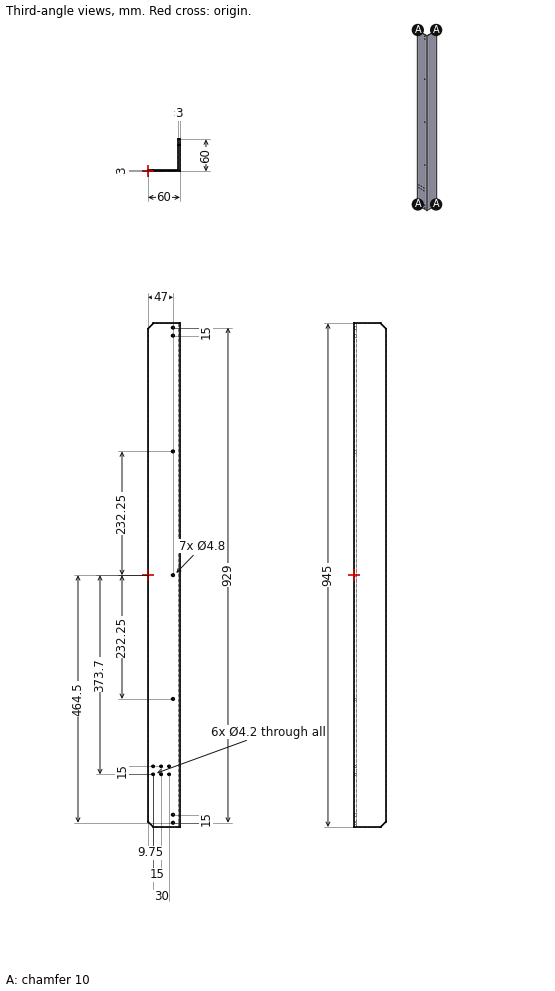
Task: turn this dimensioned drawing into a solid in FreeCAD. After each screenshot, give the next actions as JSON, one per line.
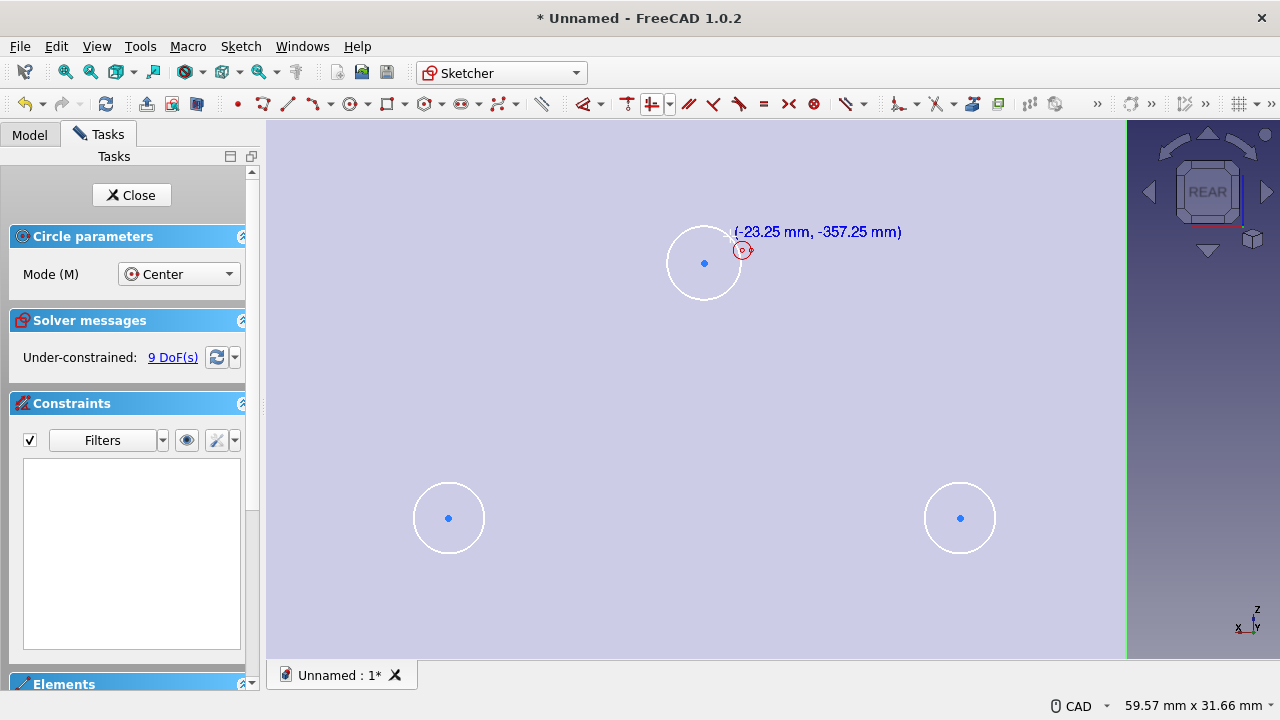
{"action": "left_click", "coordinate": [960, 262]}
{"action": "left_click", "coordinate": [985, 236]}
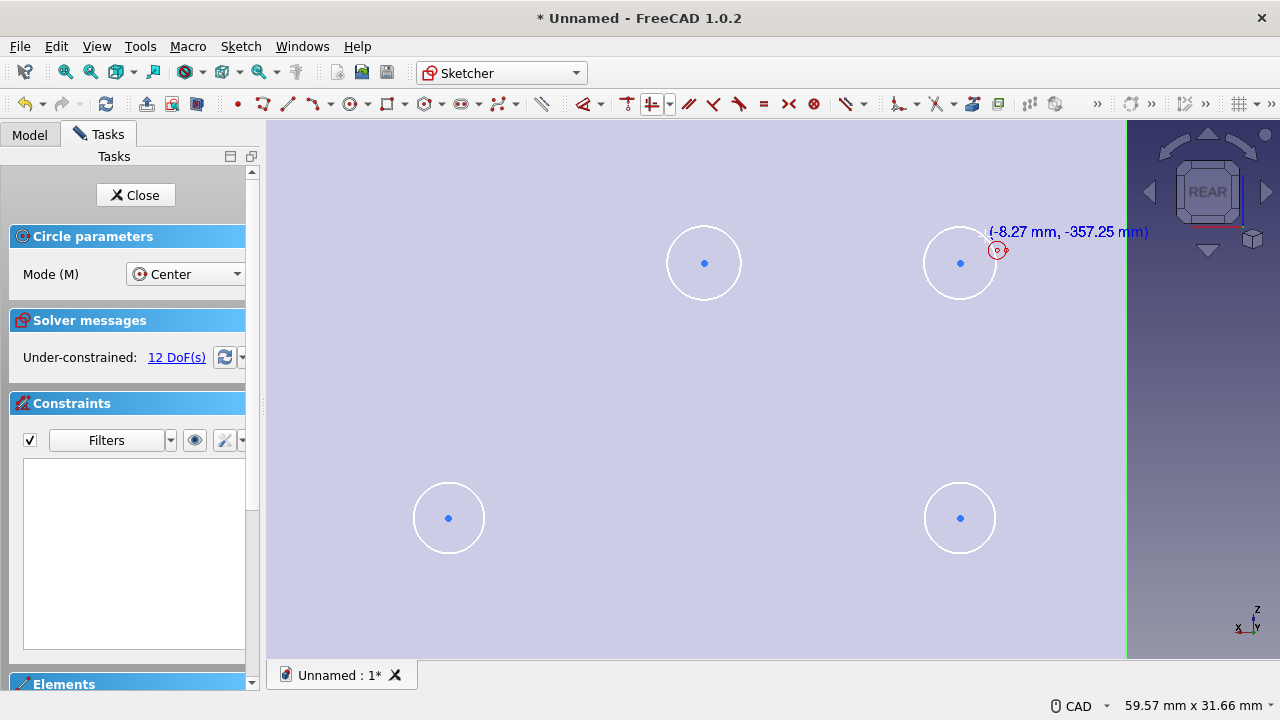
{"action": "left_click", "coordinate": [449, 262]}
{"action": "left_click", "coordinate": [474, 236]}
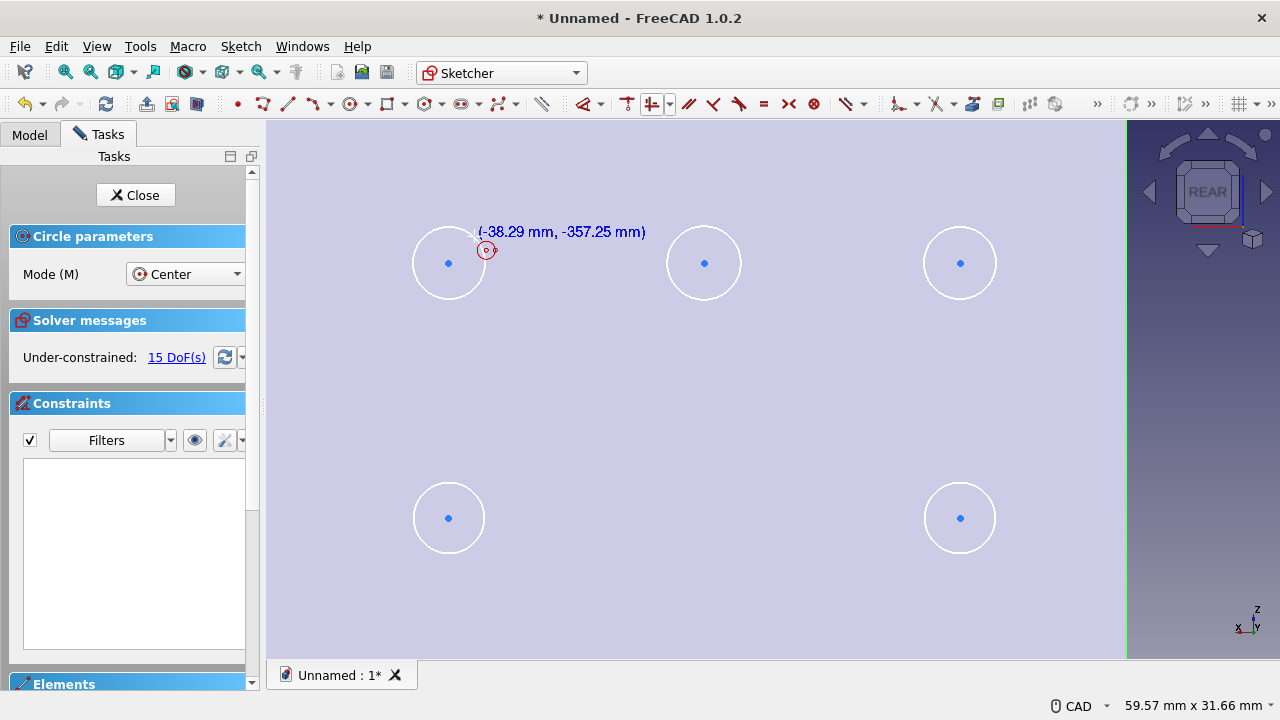
{"action": "left_click", "coordinate": [704, 517]}
{"action": "left_click", "coordinate": [730, 492]}
{"action": "key", "text": "Escape"}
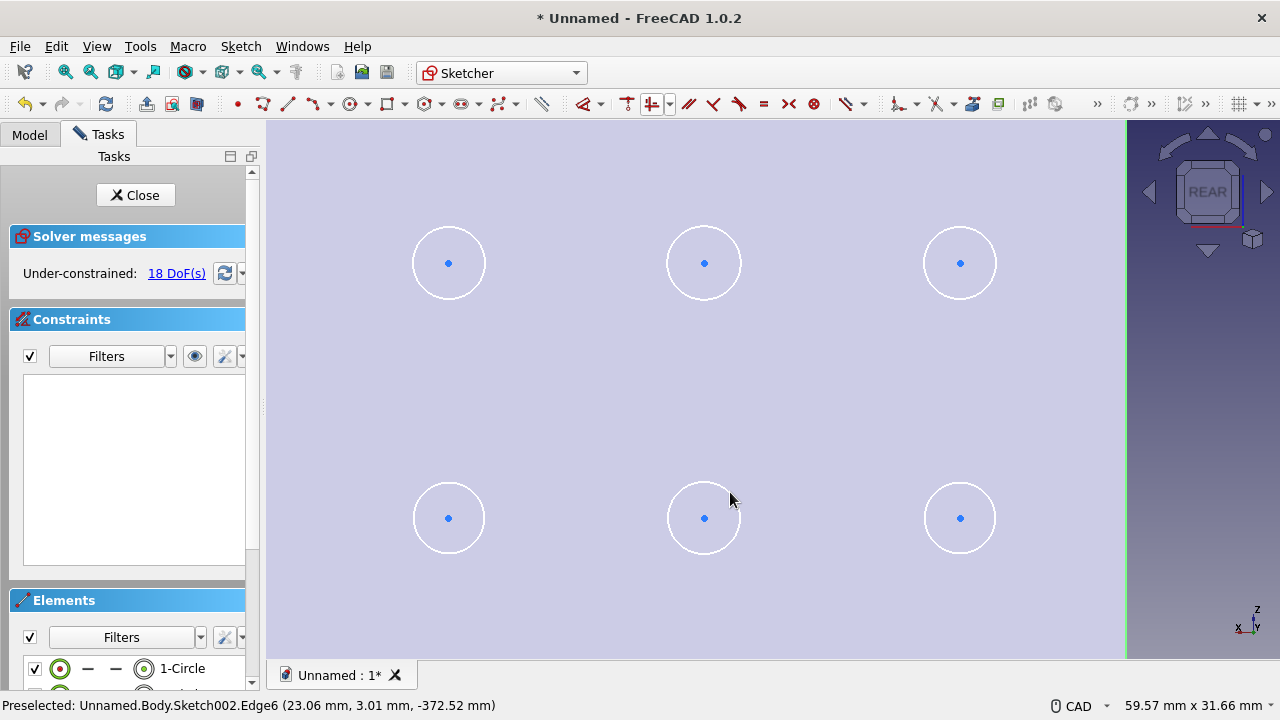
{"action": "left_click", "coordinate": [985, 493]}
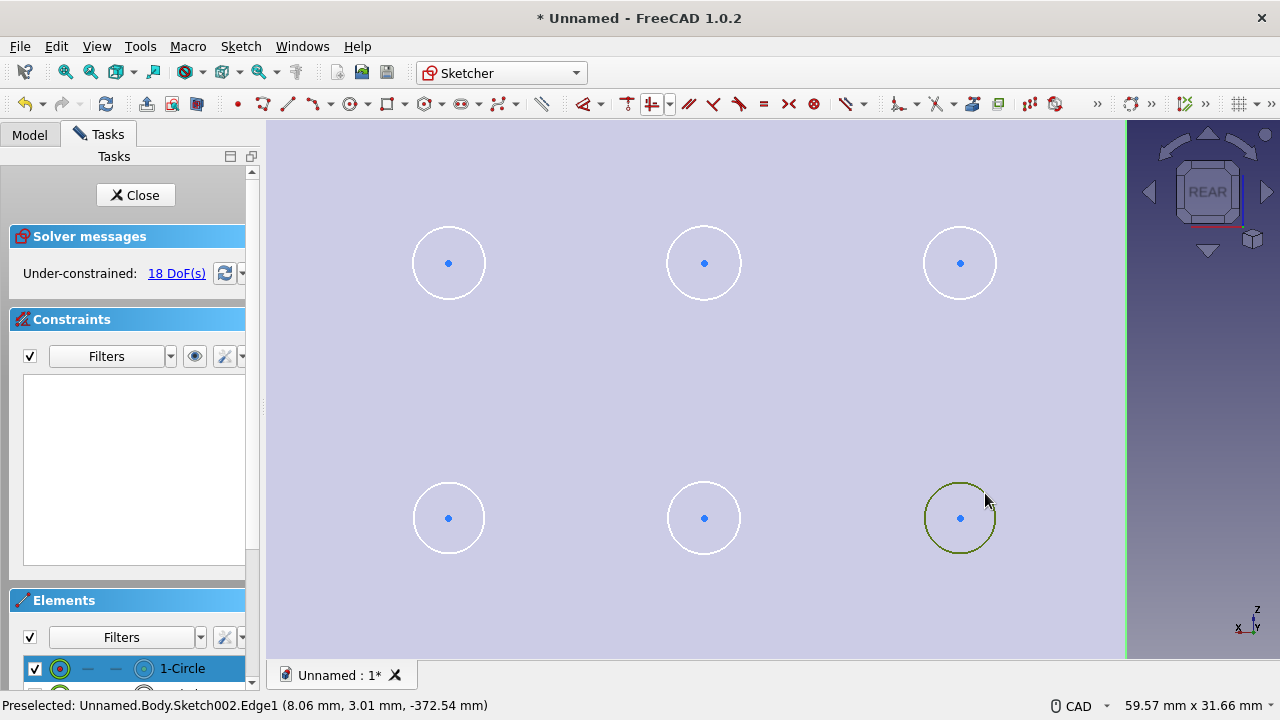
{"action": "left_click", "coordinate": [474, 493]}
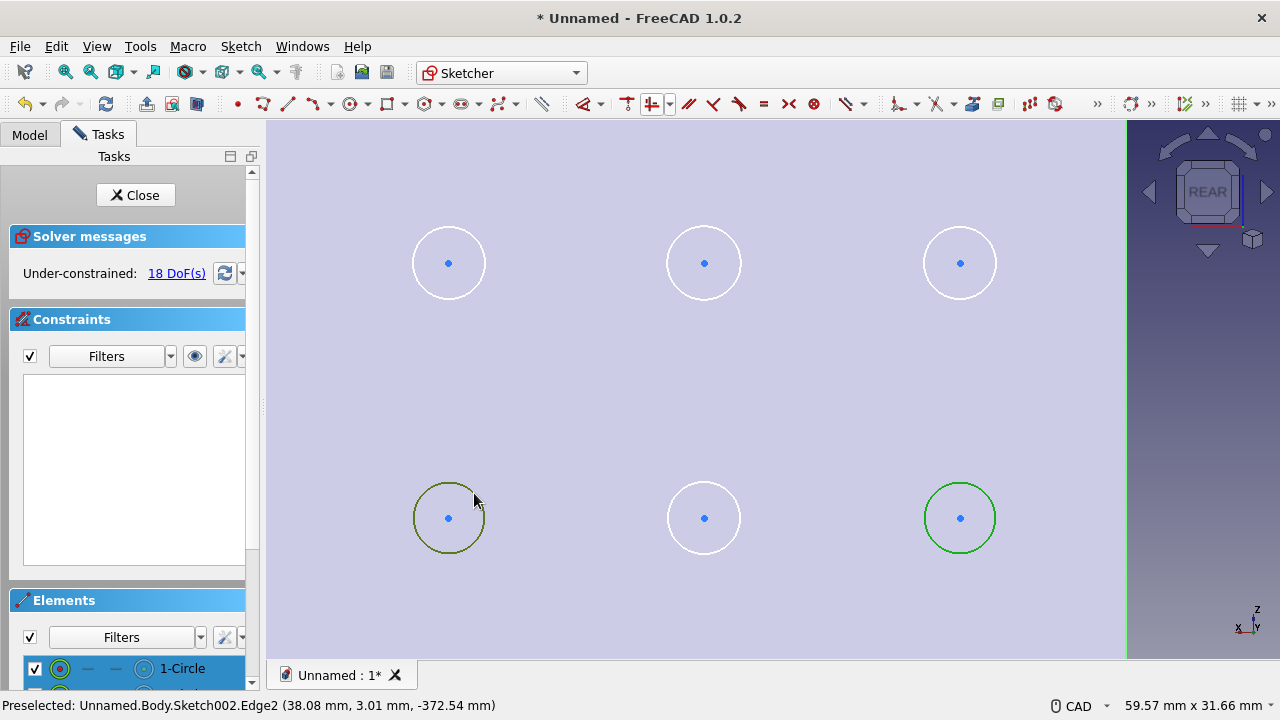
{"action": "left_click", "coordinate": [730, 237]}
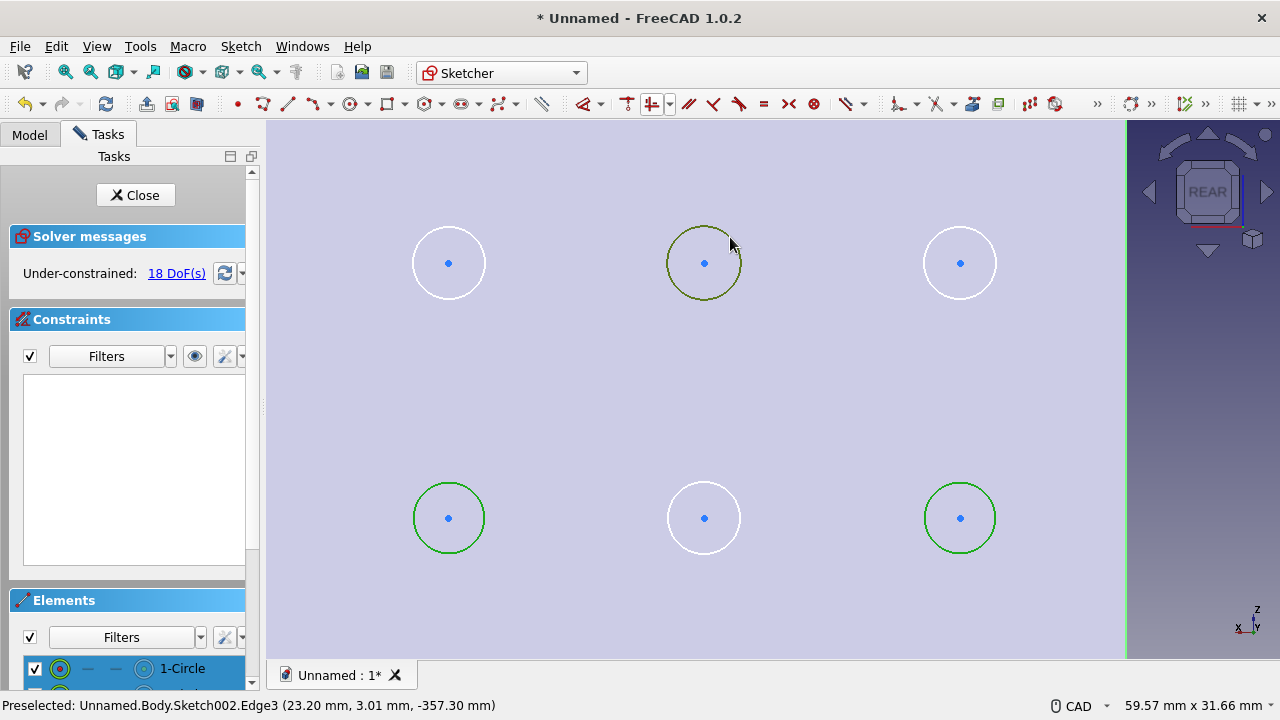
{"action": "left_click", "coordinate": [985, 237]}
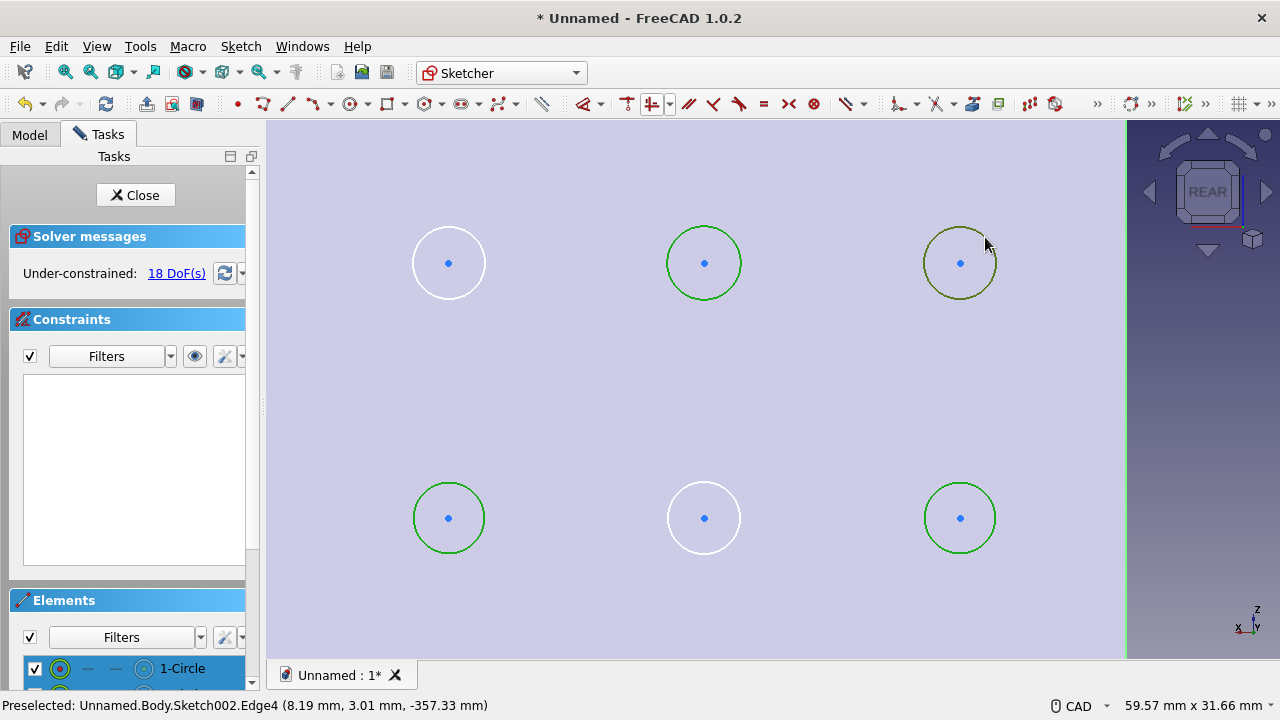
{"action": "left_click", "coordinate": [474, 237]}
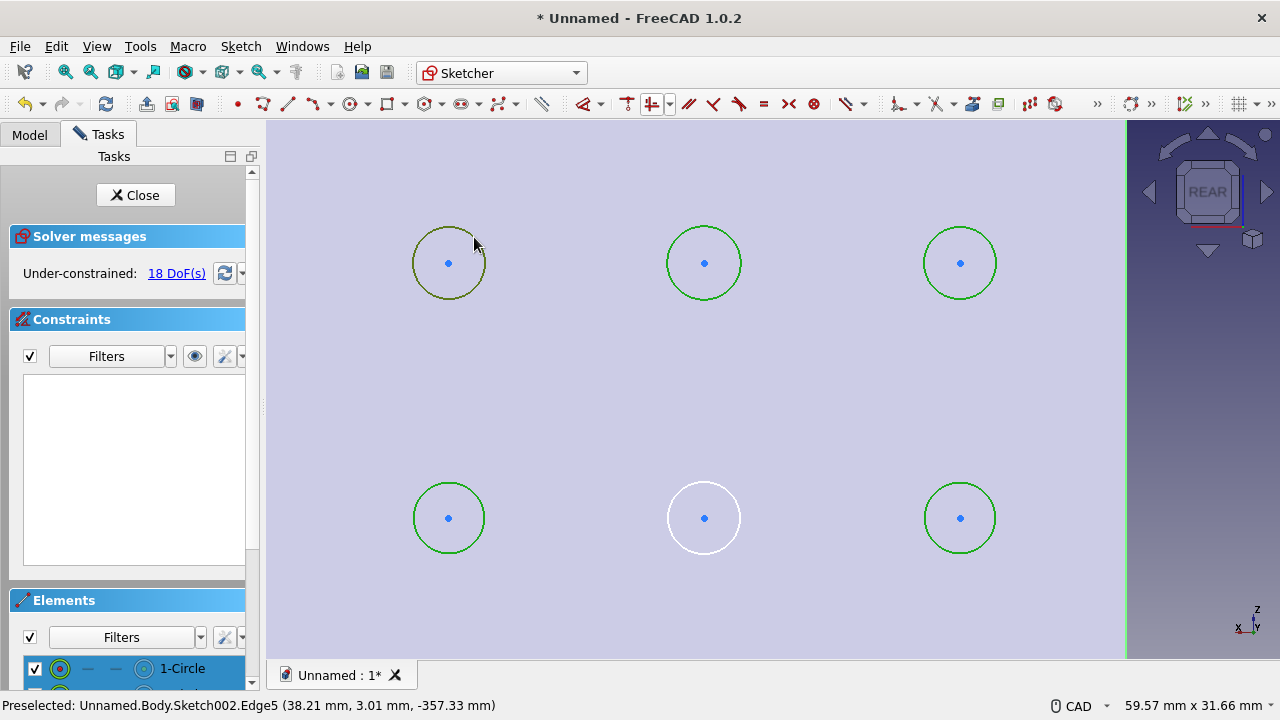
{"action": "left_click", "coordinate": [729, 492]}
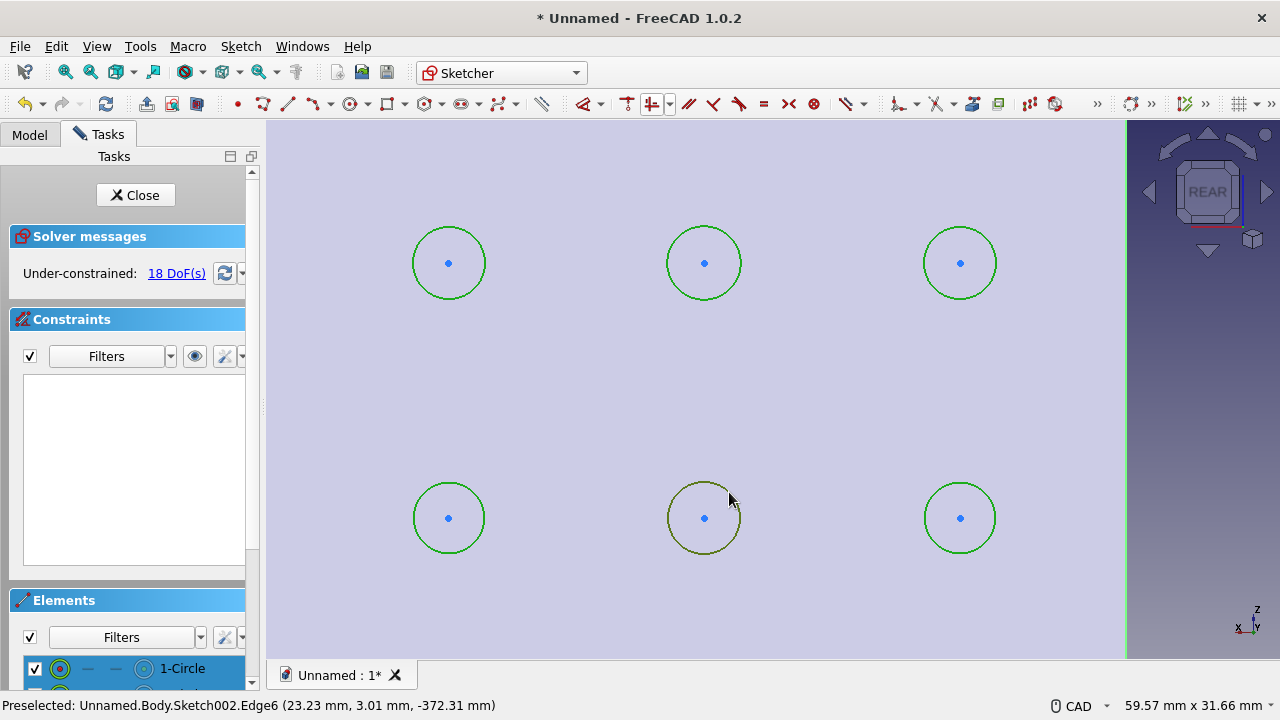
{"action": "left_click", "coordinate": [764, 104]}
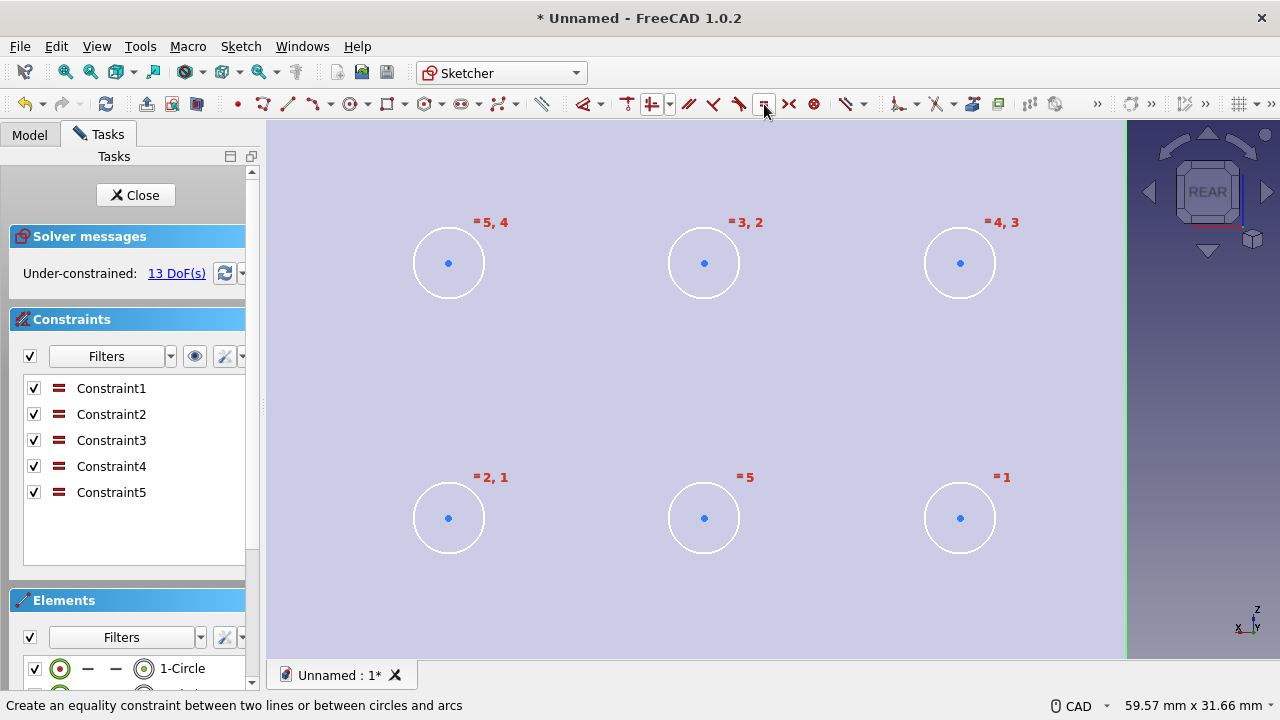
{"action": "left_click", "coordinate": [960, 518]}